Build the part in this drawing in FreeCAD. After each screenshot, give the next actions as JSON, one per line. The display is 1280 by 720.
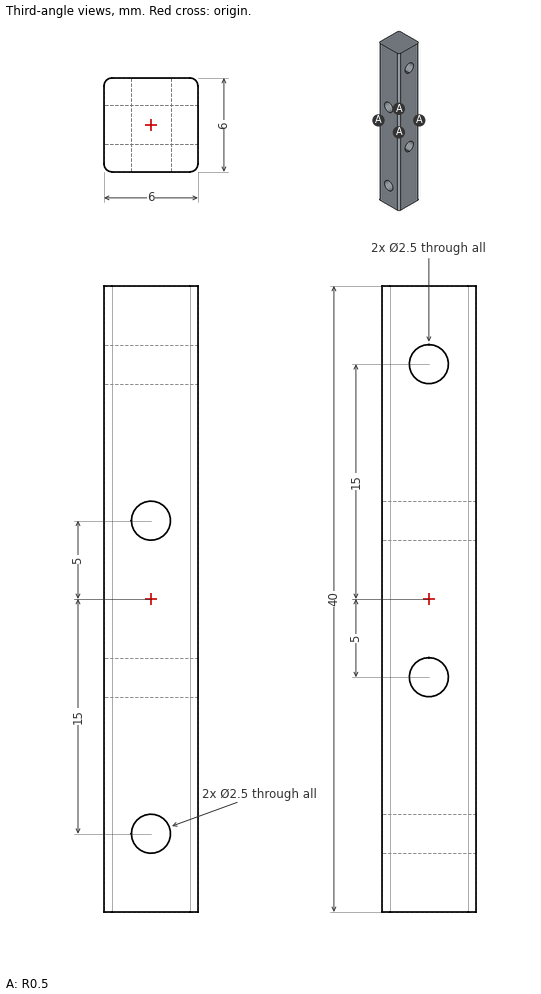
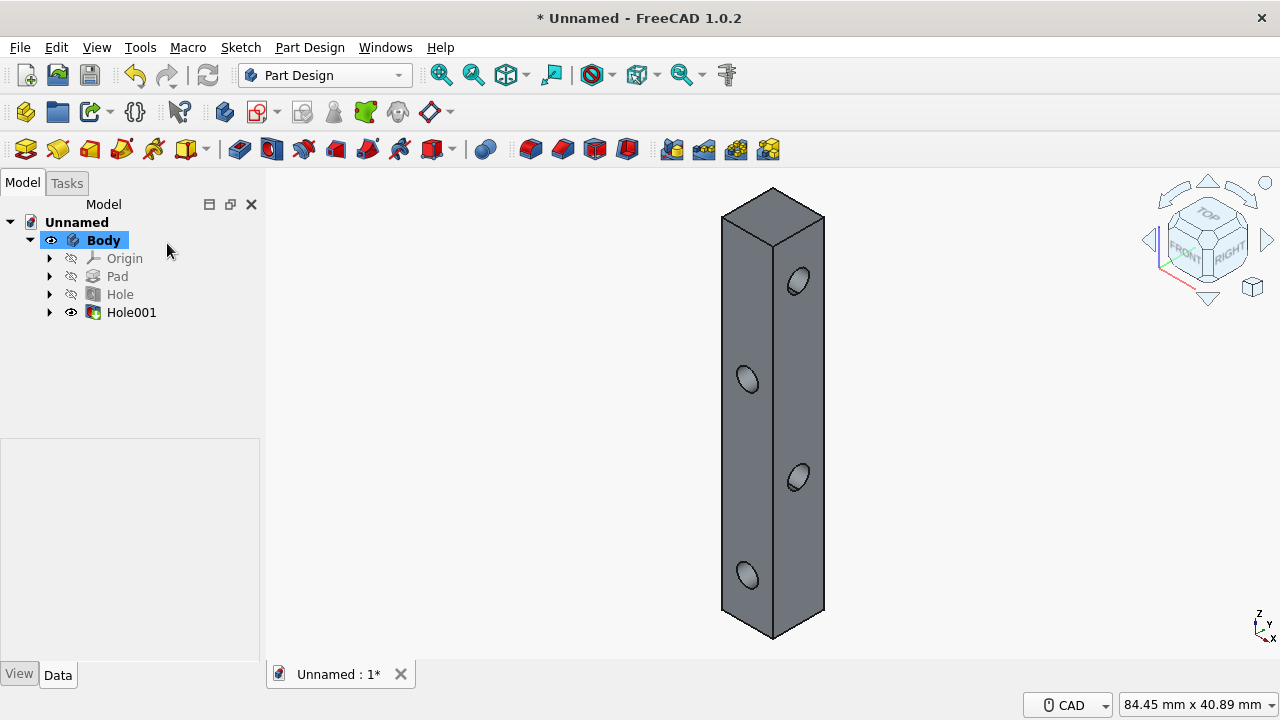
{"action": "left_click", "coordinate": [773, 442]}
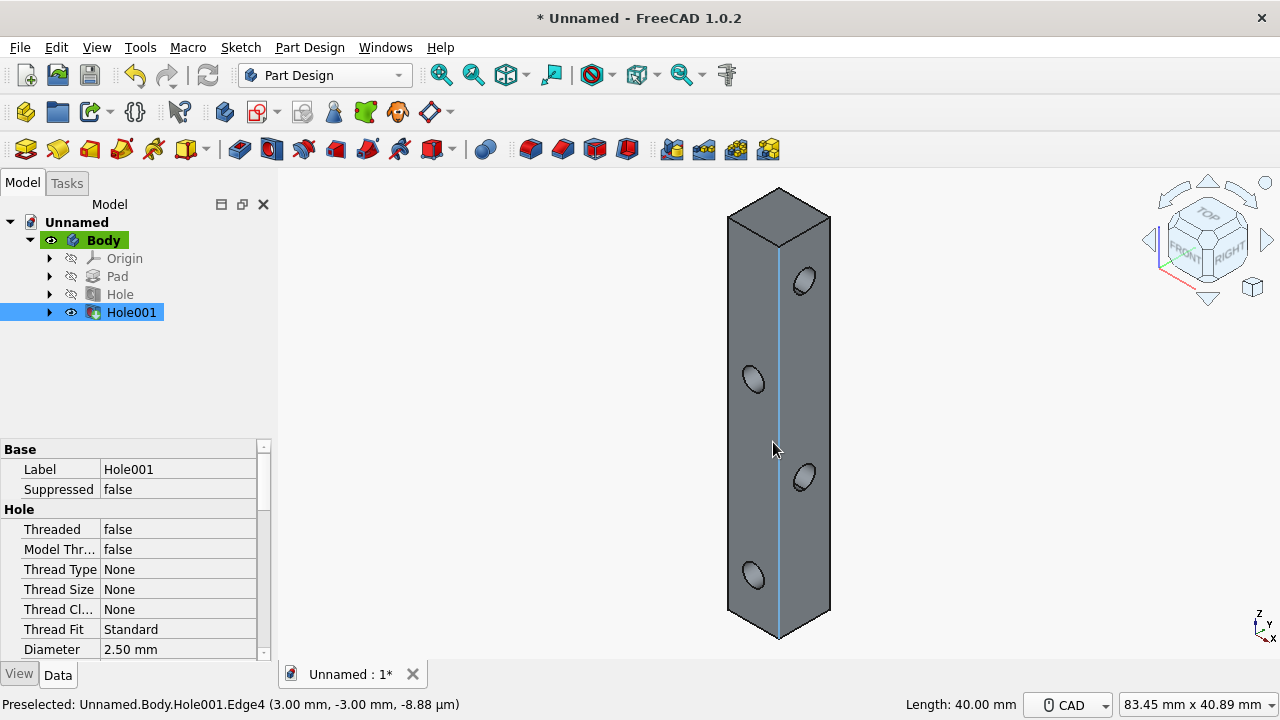
{"action": "key", "text": "2"}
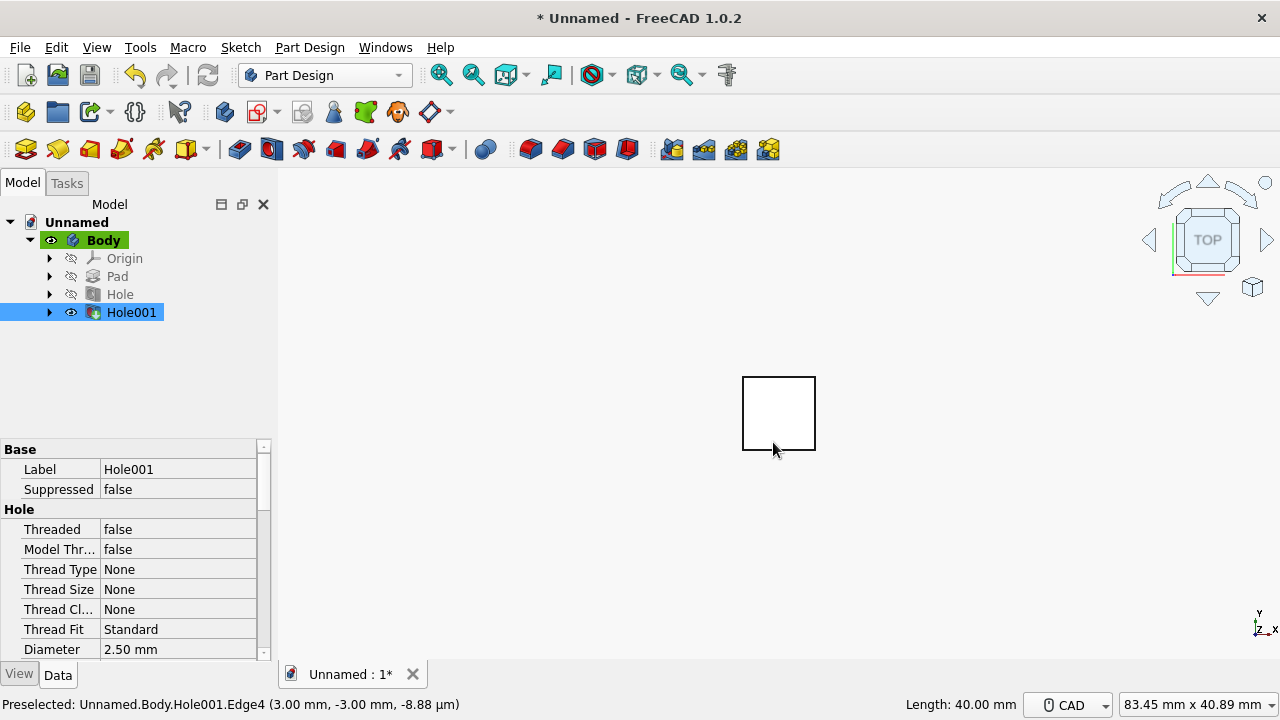
{"action": "left_click", "coordinate": [442, 76]}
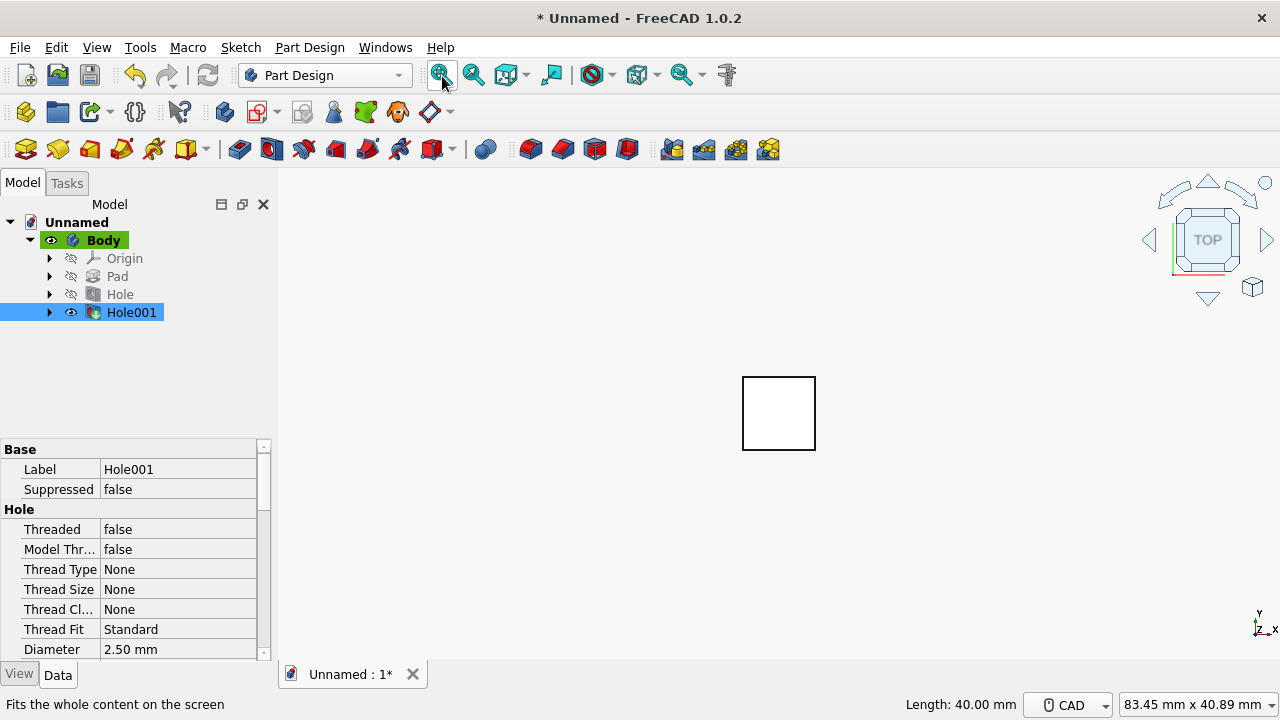
{"action": "key", "text": "0"}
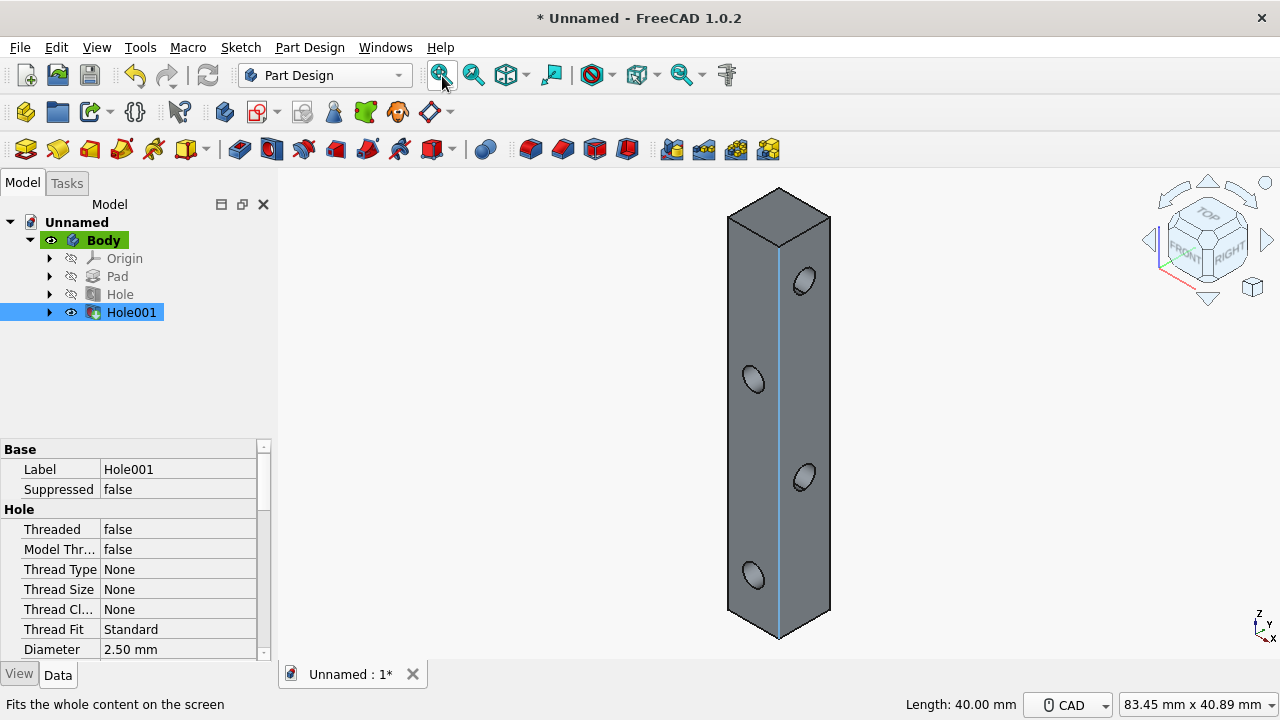
{"action": "key", "text": "1"}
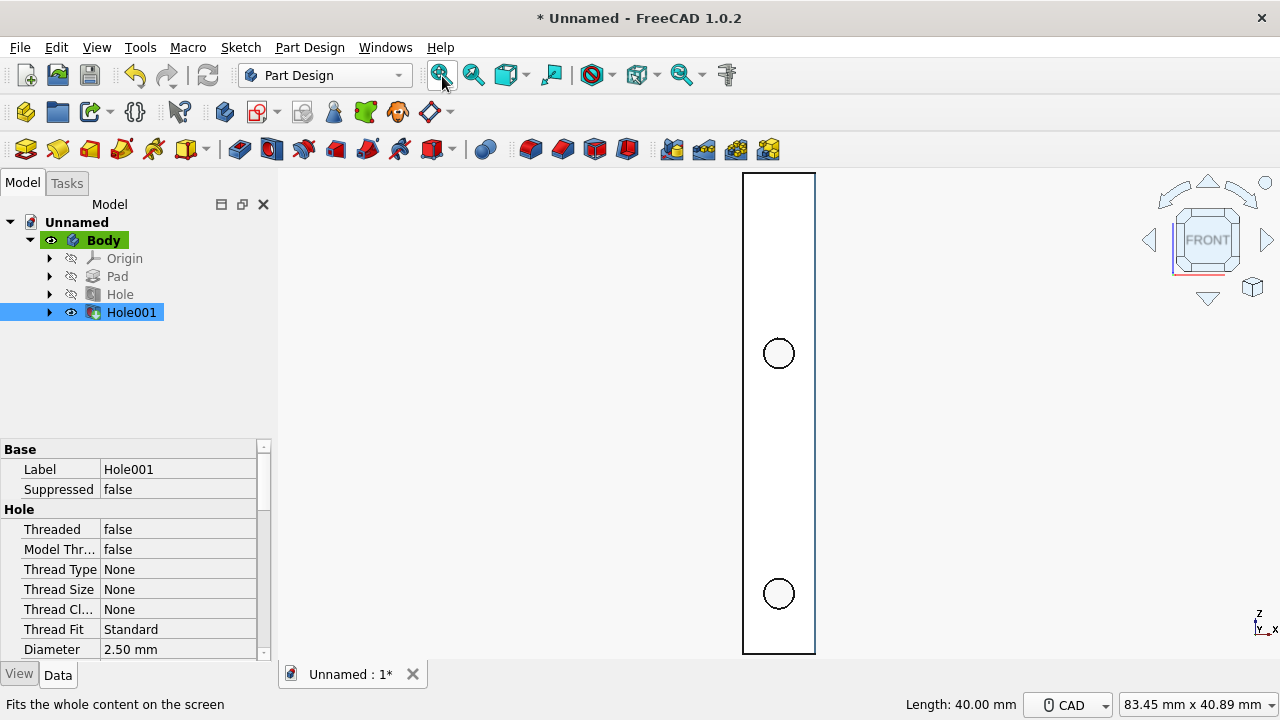
{"action": "left_click", "coordinate": [743, 413], "text": "ctrl"}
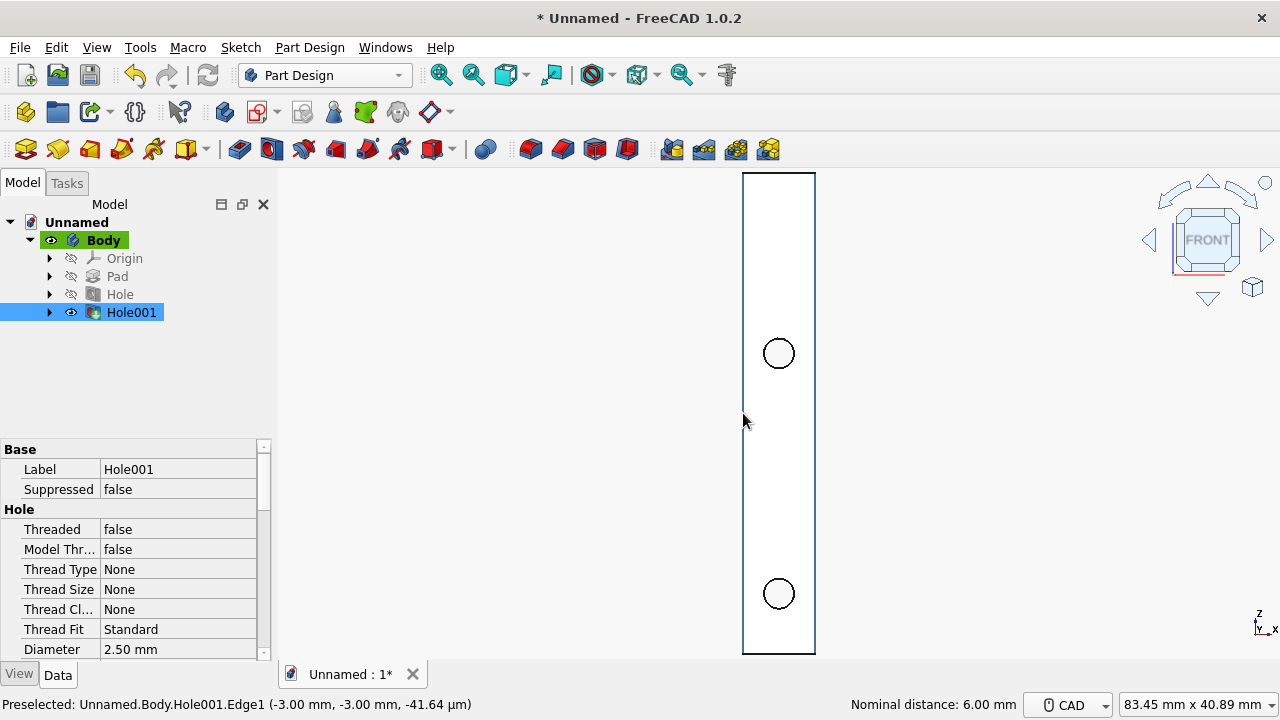
{"action": "key", "text": "3"}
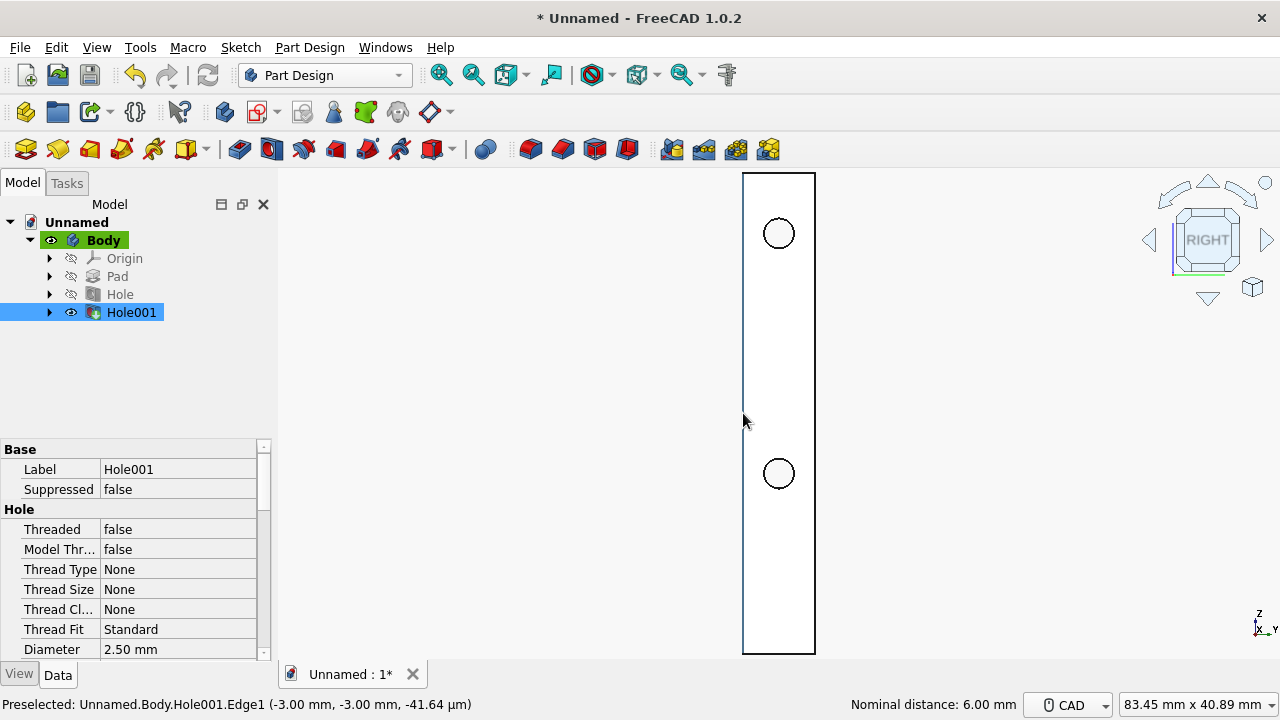
{"action": "left_click", "coordinate": [815, 413], "text": "ctrl"}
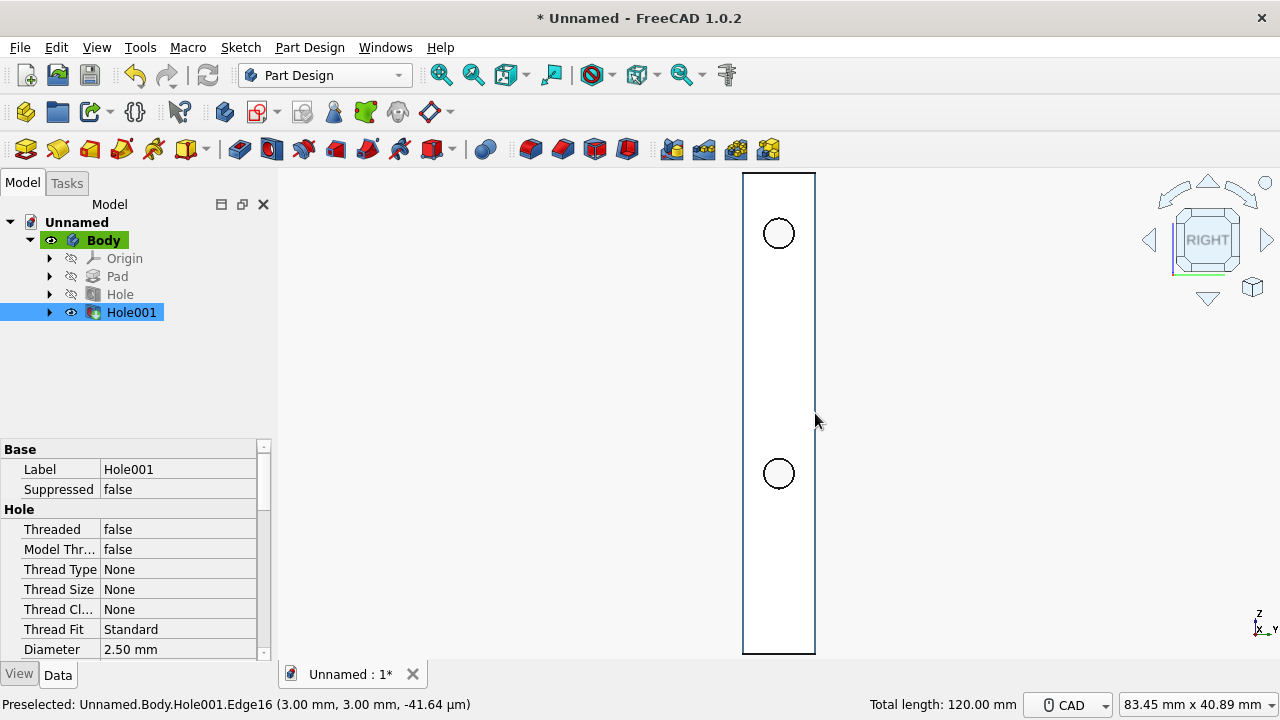
{"action": "key", "text": "5"}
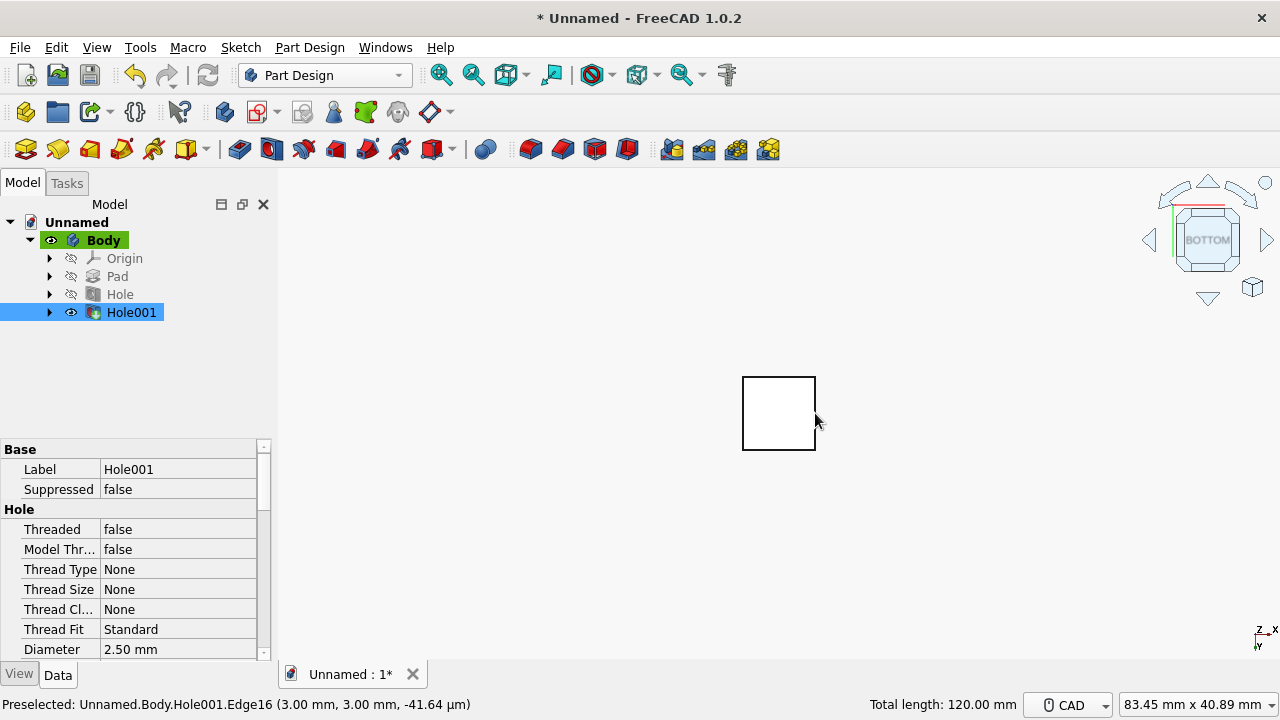
{"action": "left_click", "coordinate": [442, 76]}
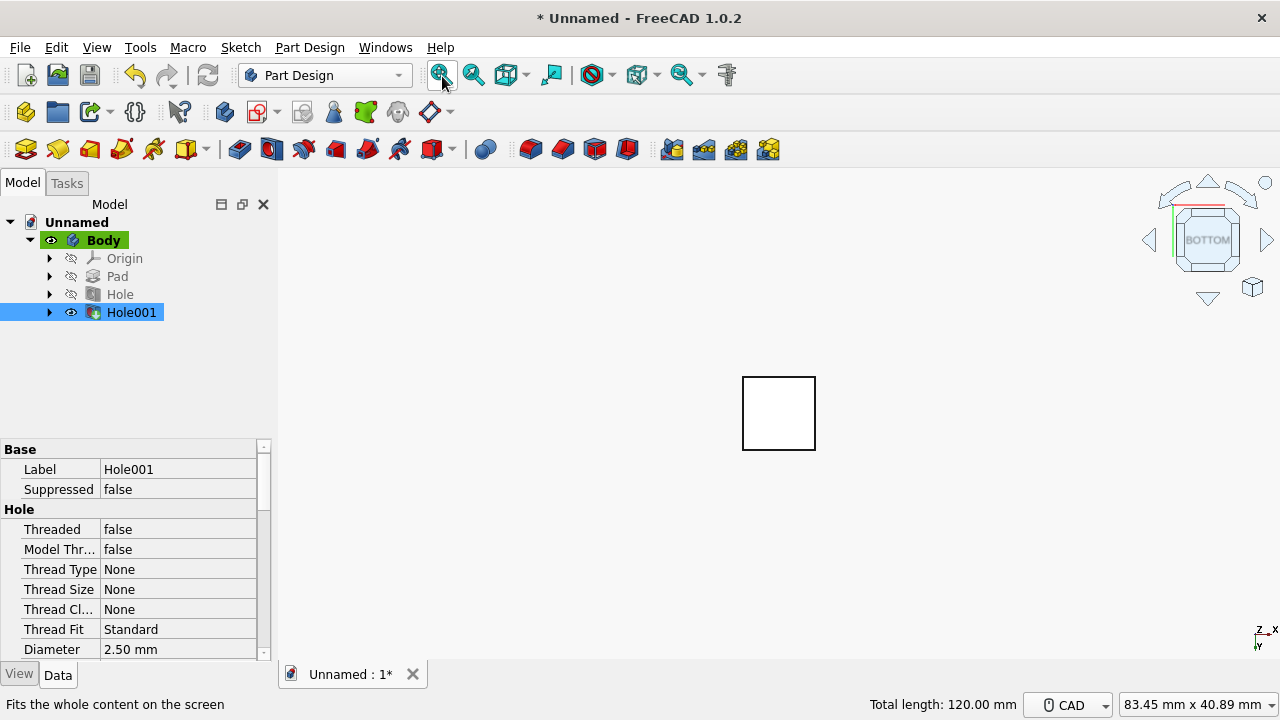
{"action": "key", "text": "4"}